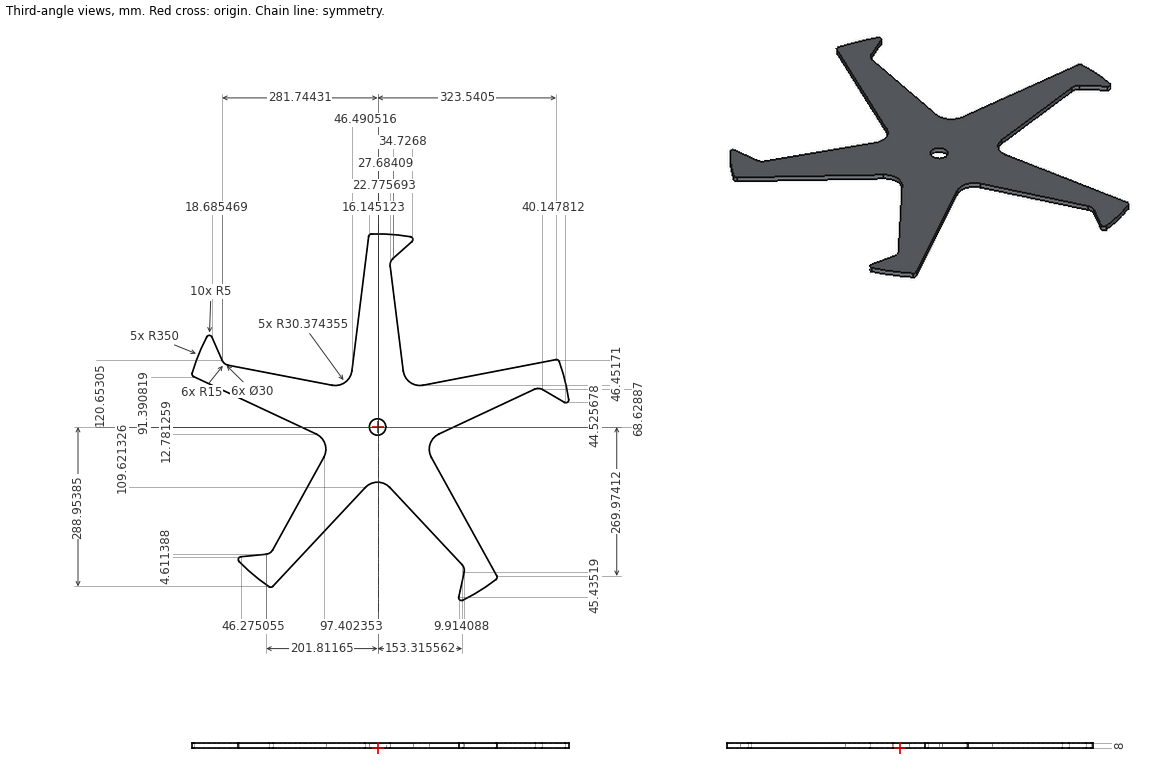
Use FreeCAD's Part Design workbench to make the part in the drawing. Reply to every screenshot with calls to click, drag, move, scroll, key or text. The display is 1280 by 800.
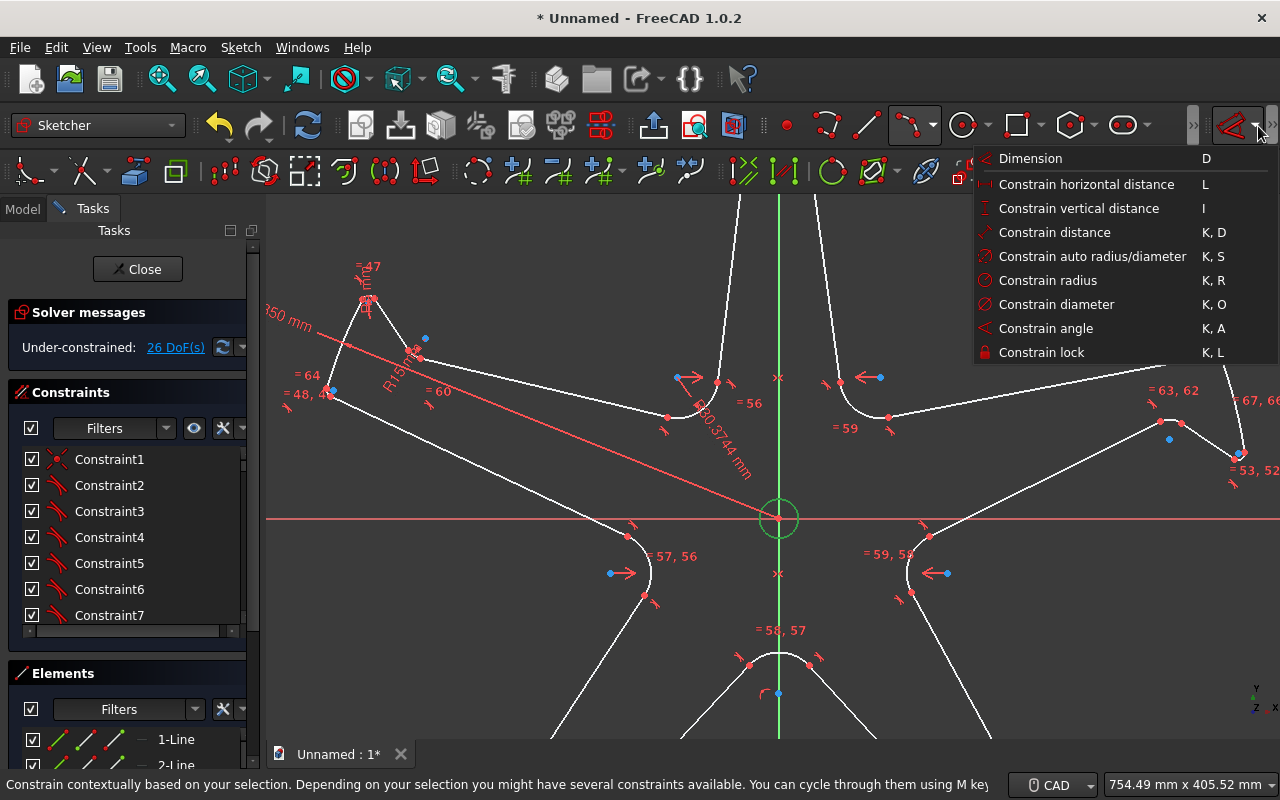
click(1126, 304)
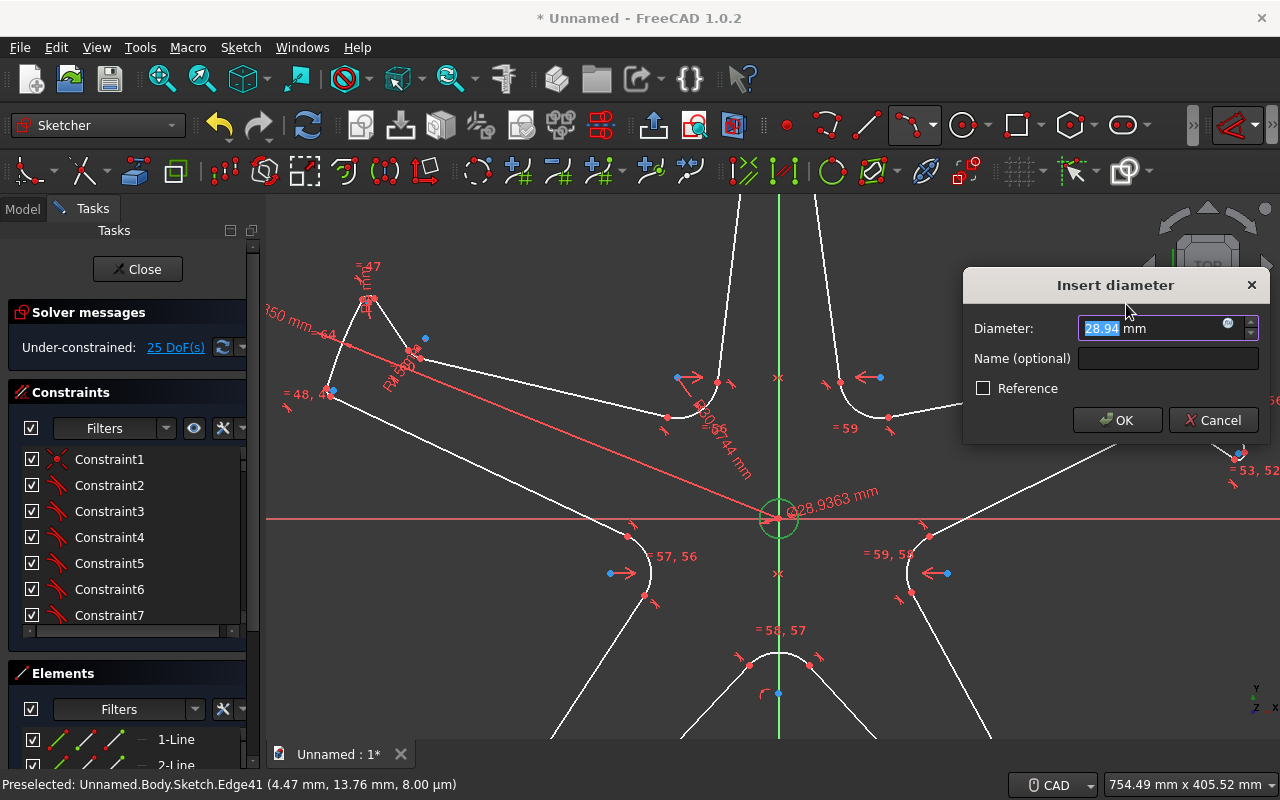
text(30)
key(Return)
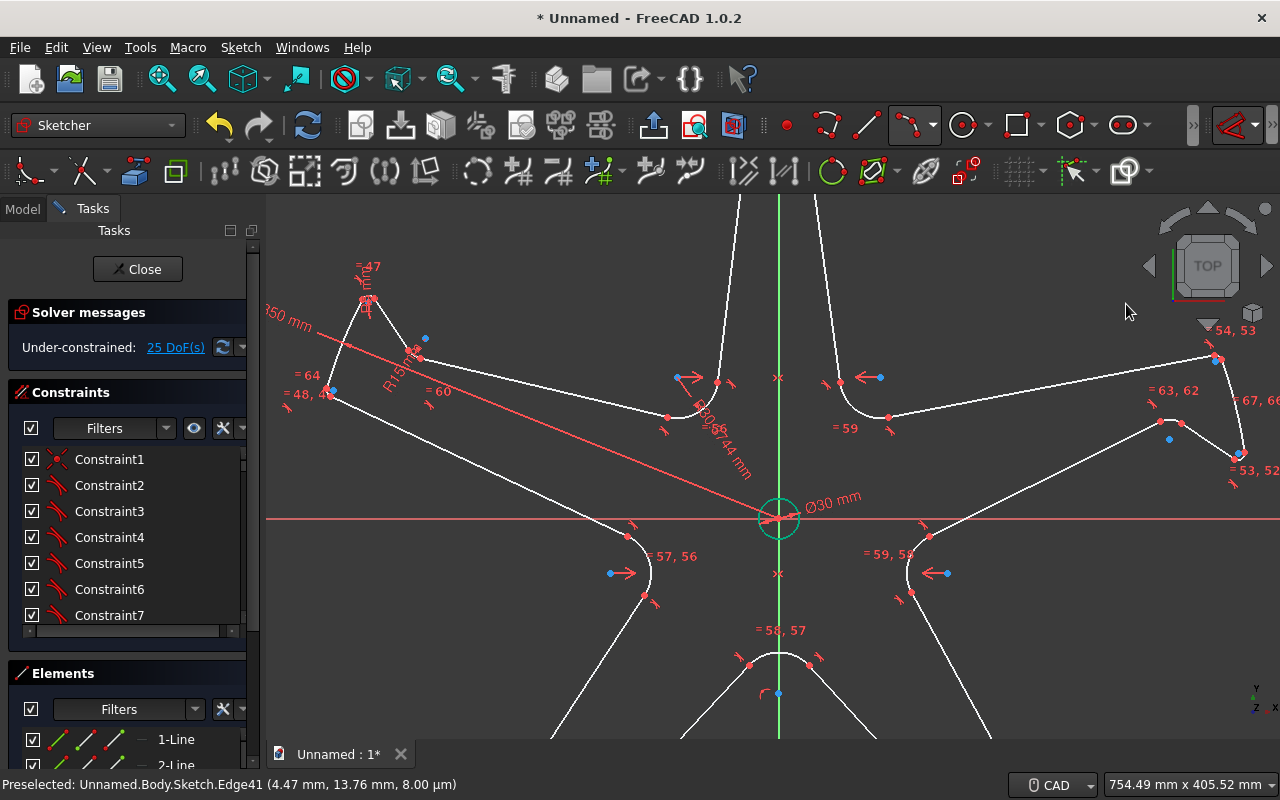
scroll(657, 450, down, 5)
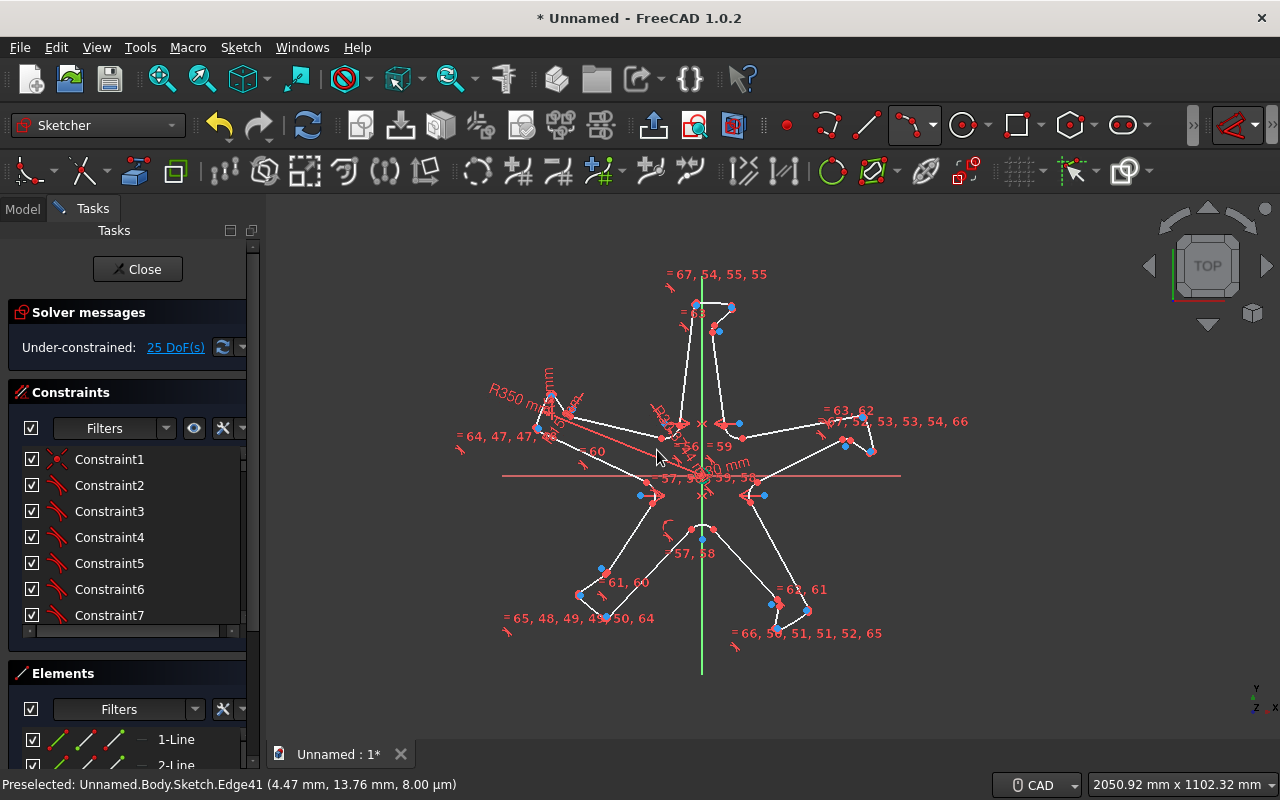
scroll(720, 321, up, 5)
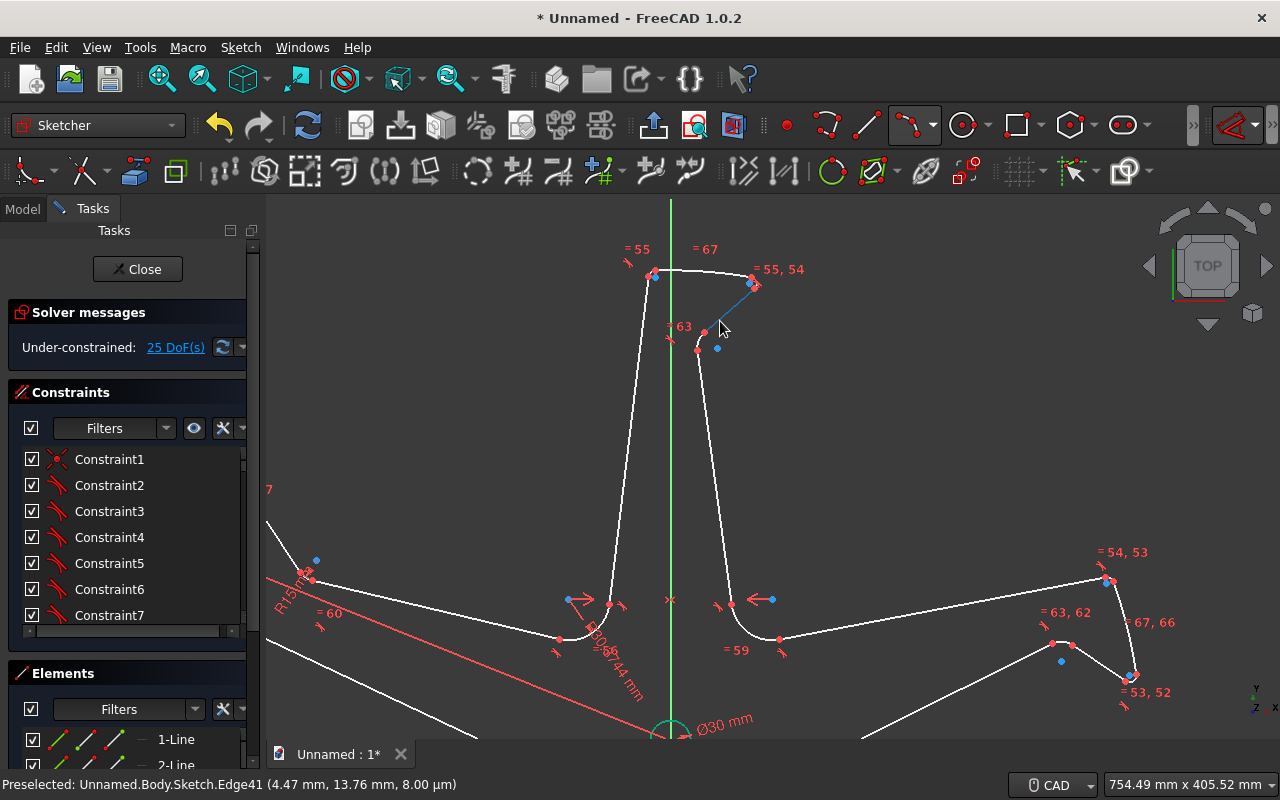
click(719, 320)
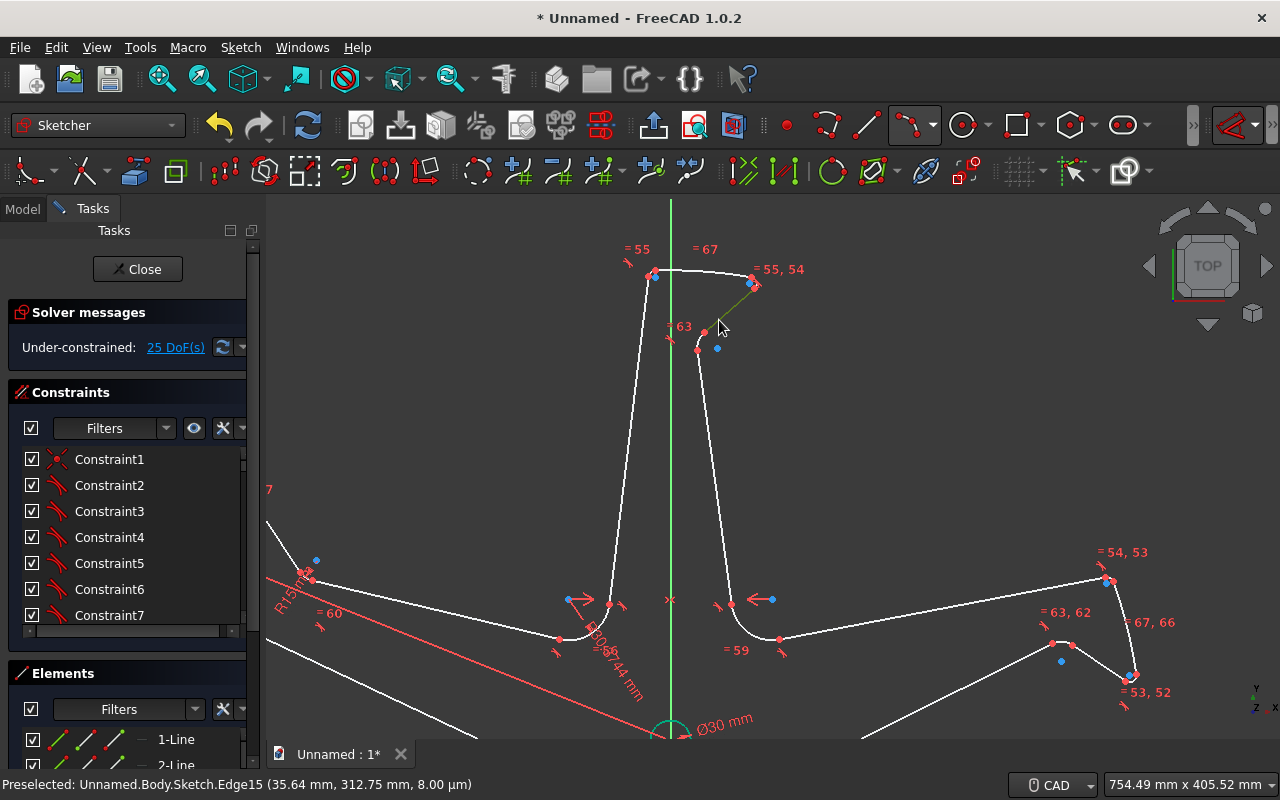
click(1258, 126)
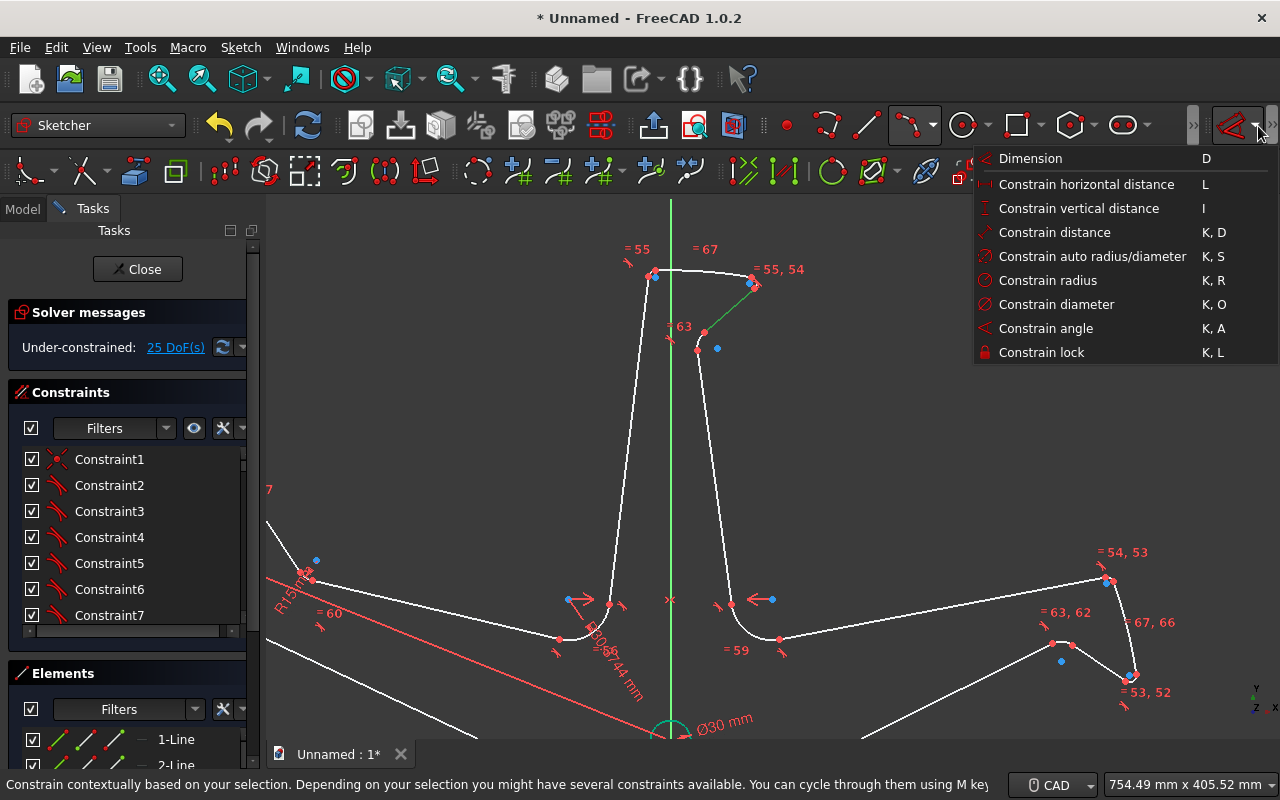
click(1126, 184)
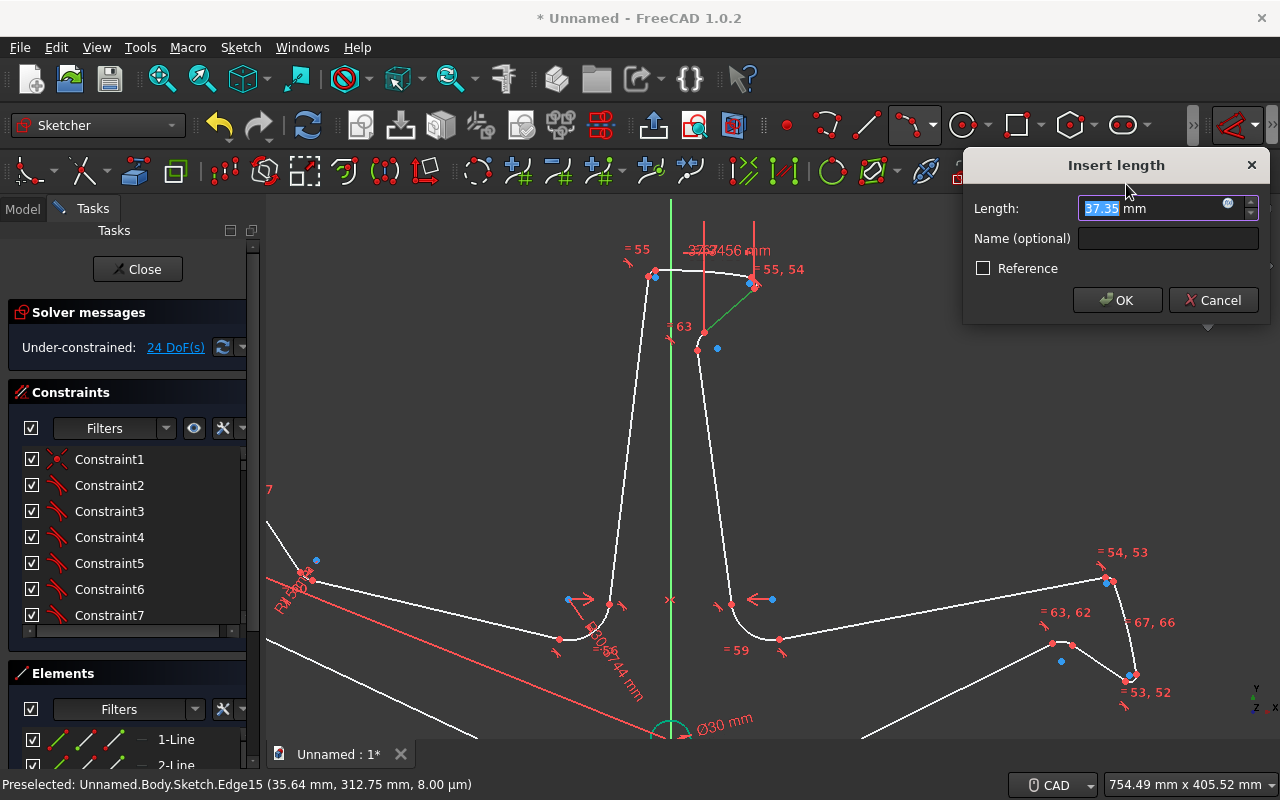
text(34.7268)
key(Return)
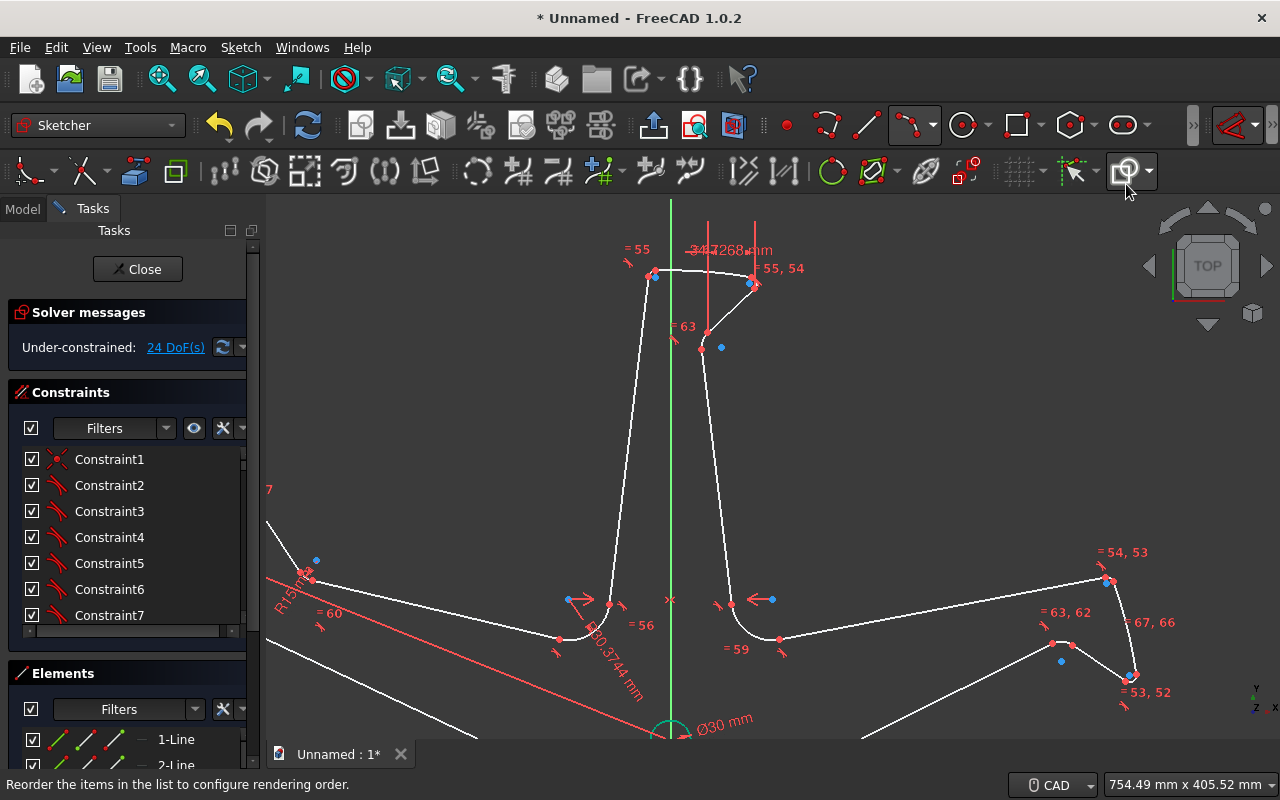
click(1052, 644)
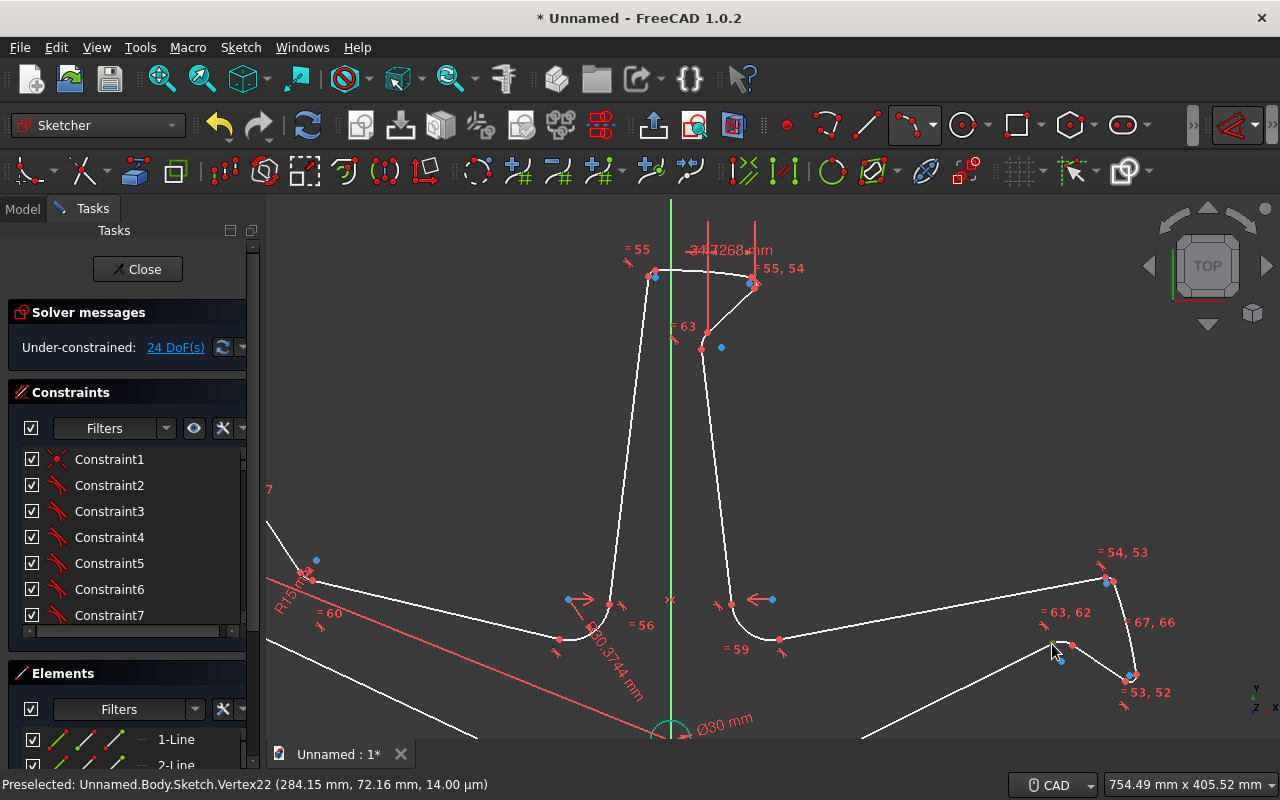
click(1258, 126)